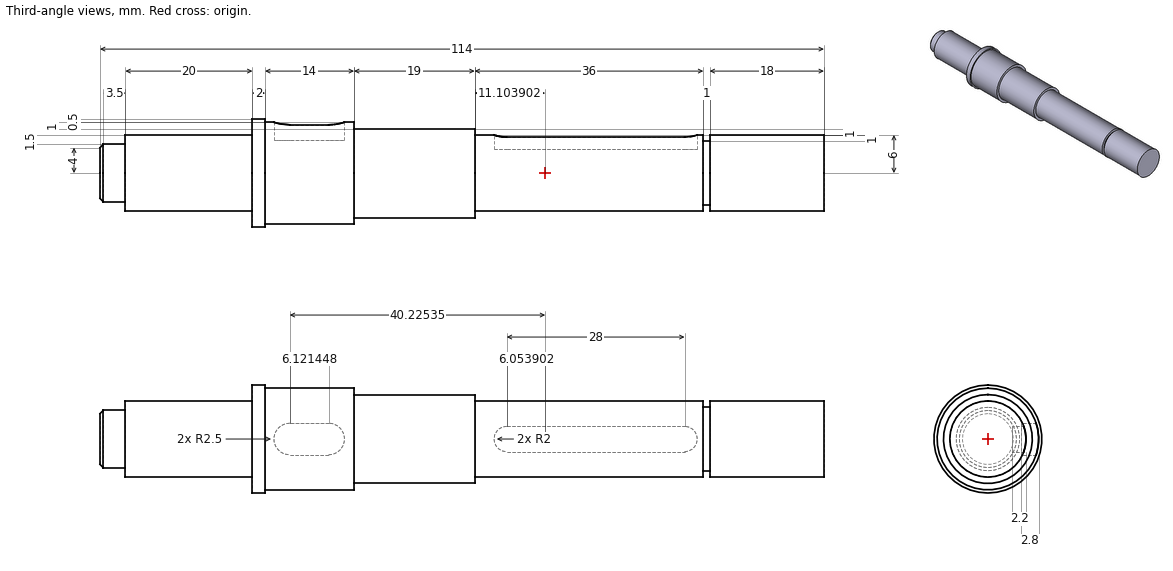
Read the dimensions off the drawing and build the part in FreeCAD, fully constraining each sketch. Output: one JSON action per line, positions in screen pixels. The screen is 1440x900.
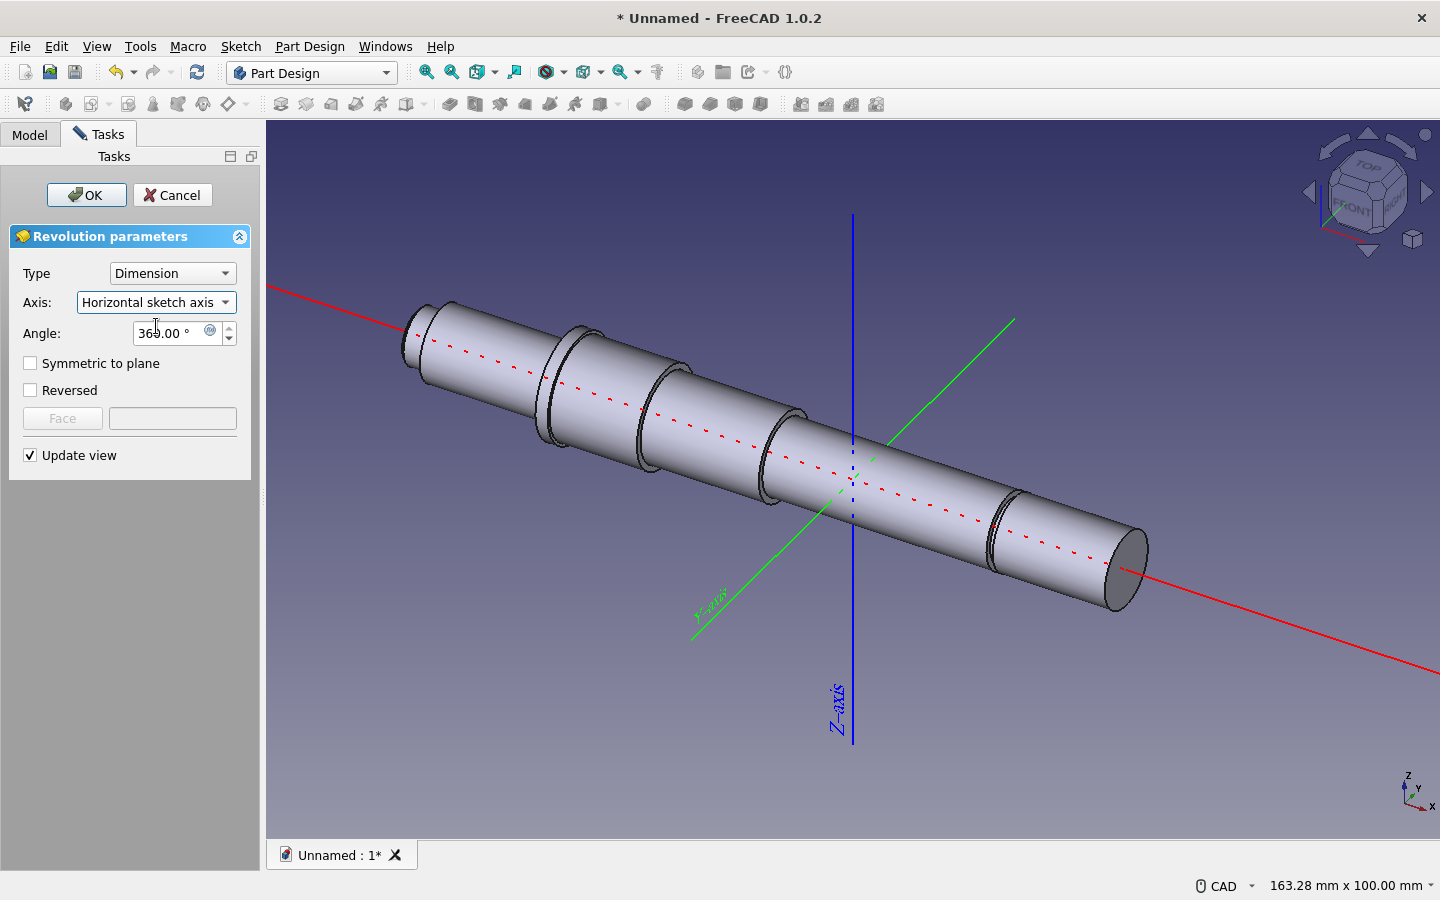
{"action": "left_click", "coordinate": [87, 195]}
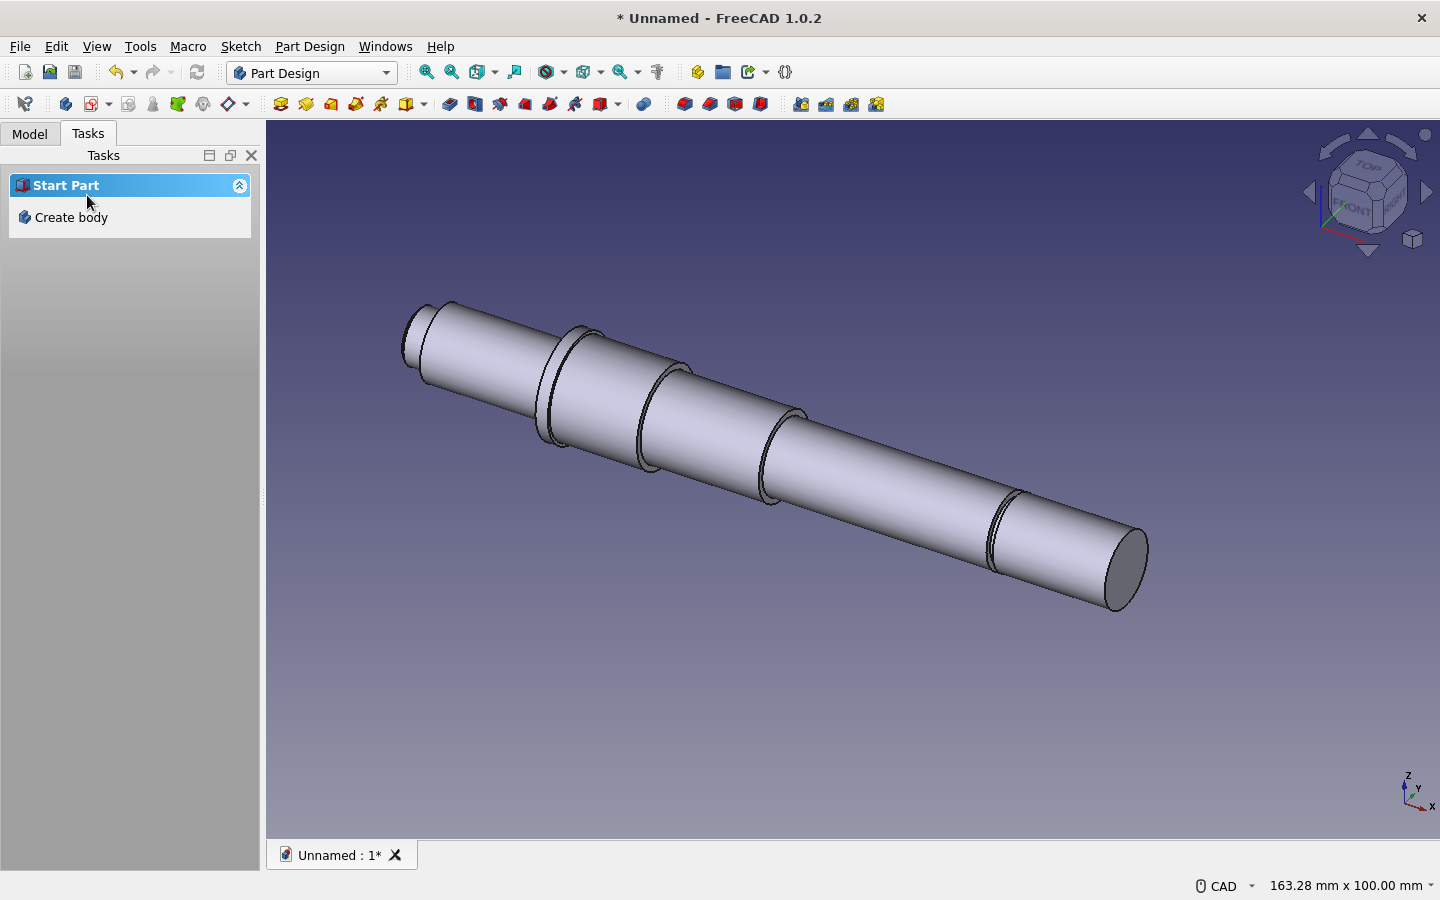
{"action": "left_click", "coordinate": [30, 134]}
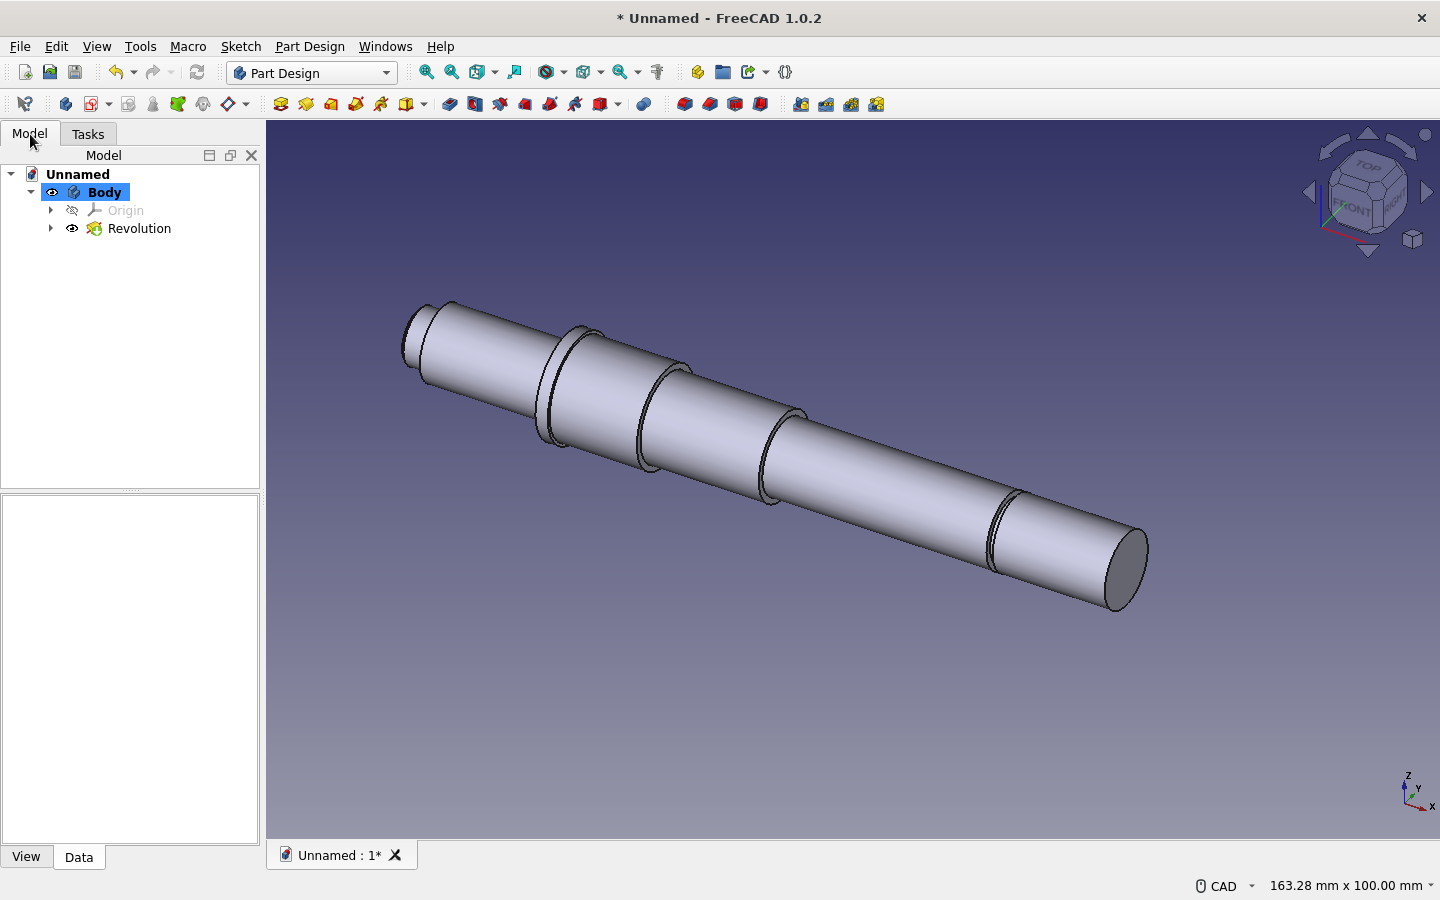
{"action": "left_click", "coordinate": [51, 210]}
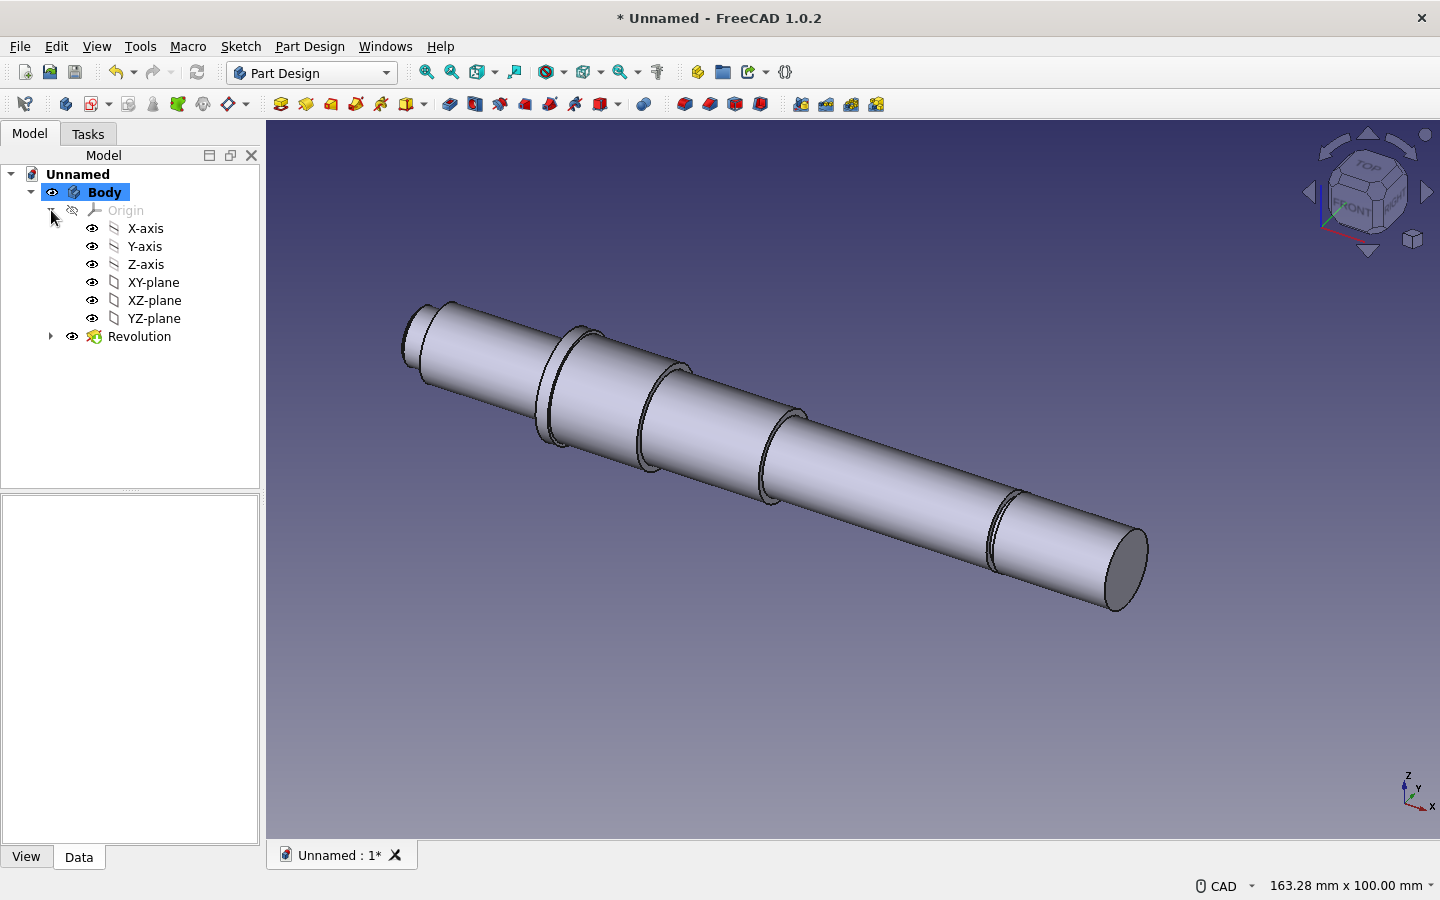
{"action": "left_click", "coordinate": [137, 300]}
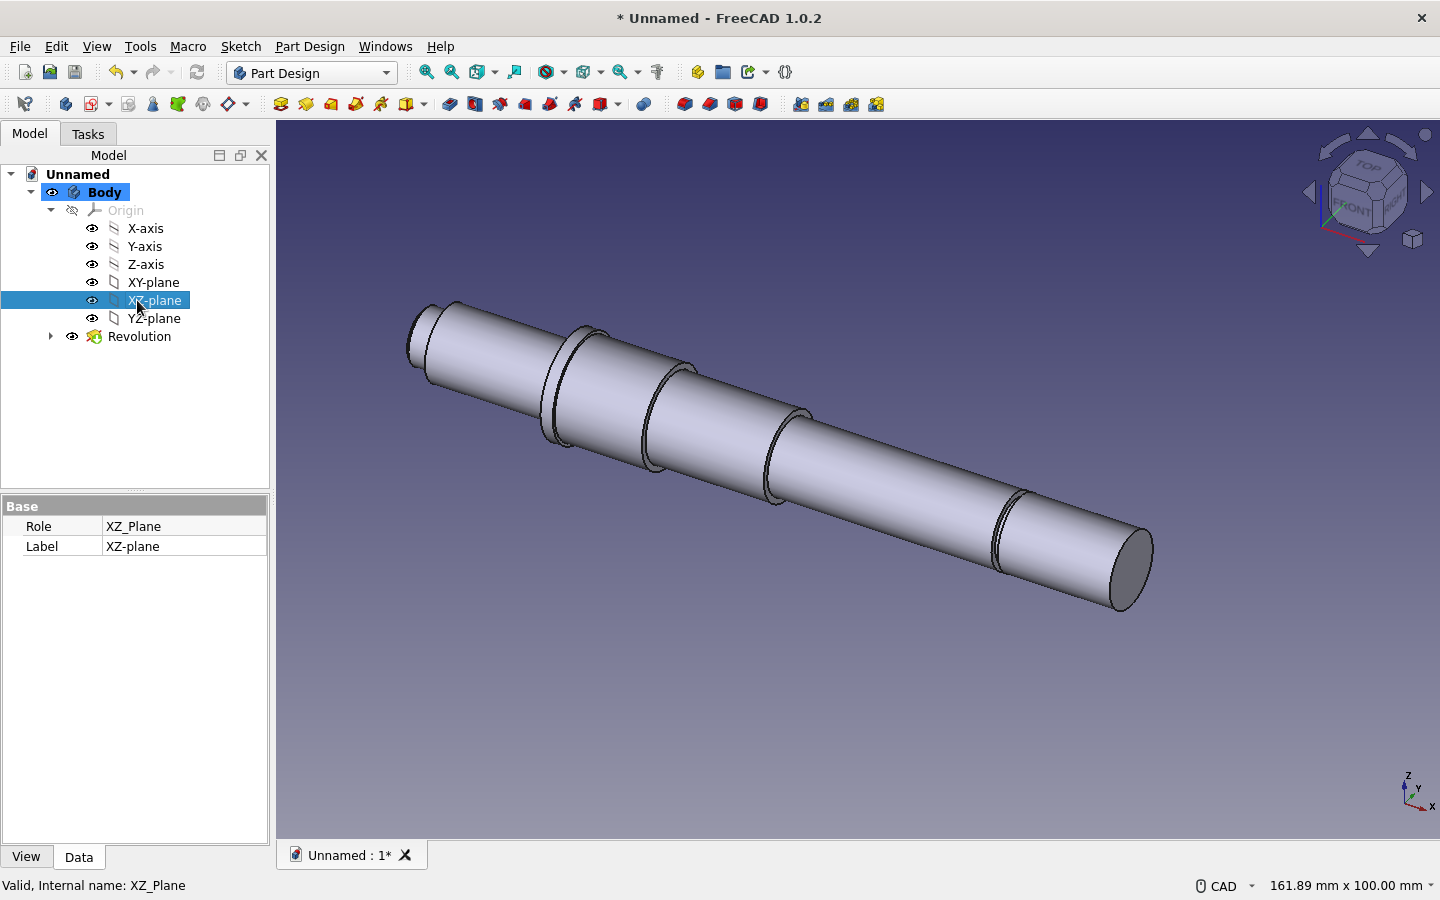
{"action": "left_click", "coordinate": [228, 104]}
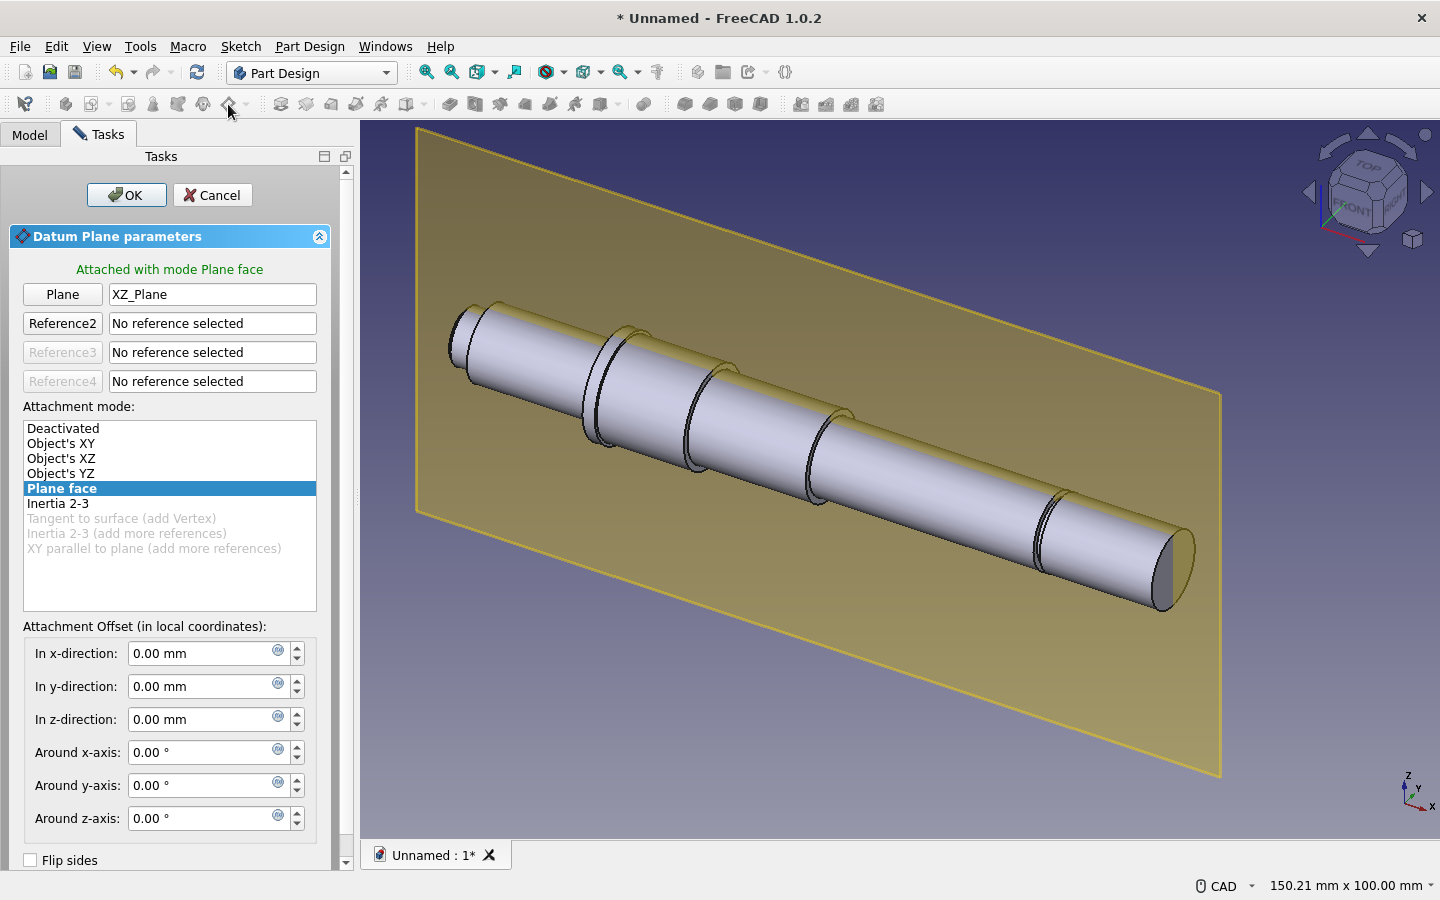
{"action": "triple_click", "coordinate": [210, 720]}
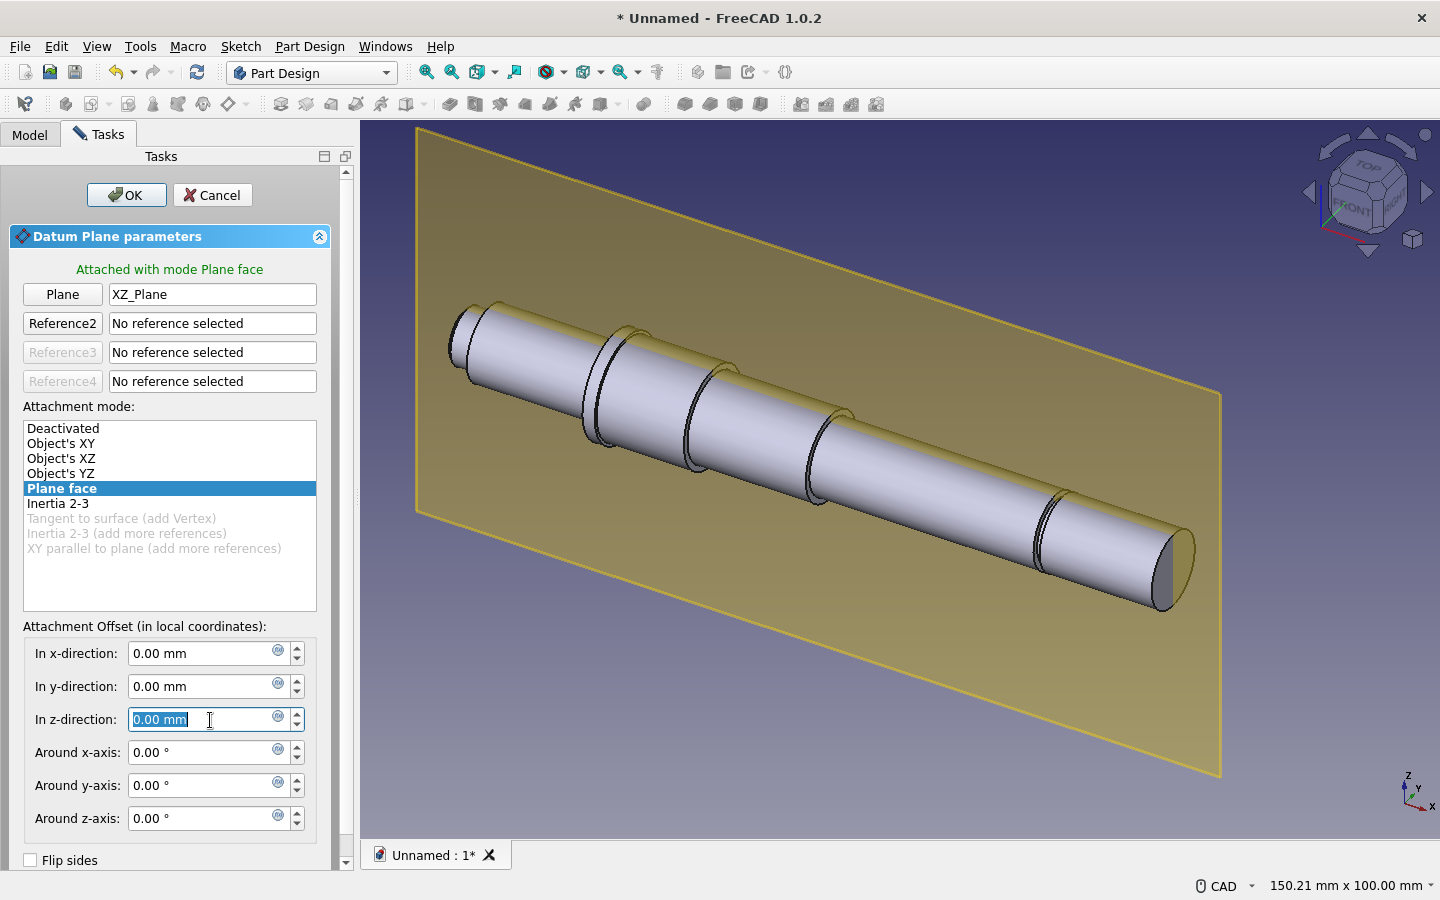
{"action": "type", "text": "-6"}
{"action": "key", "text": "Tab"}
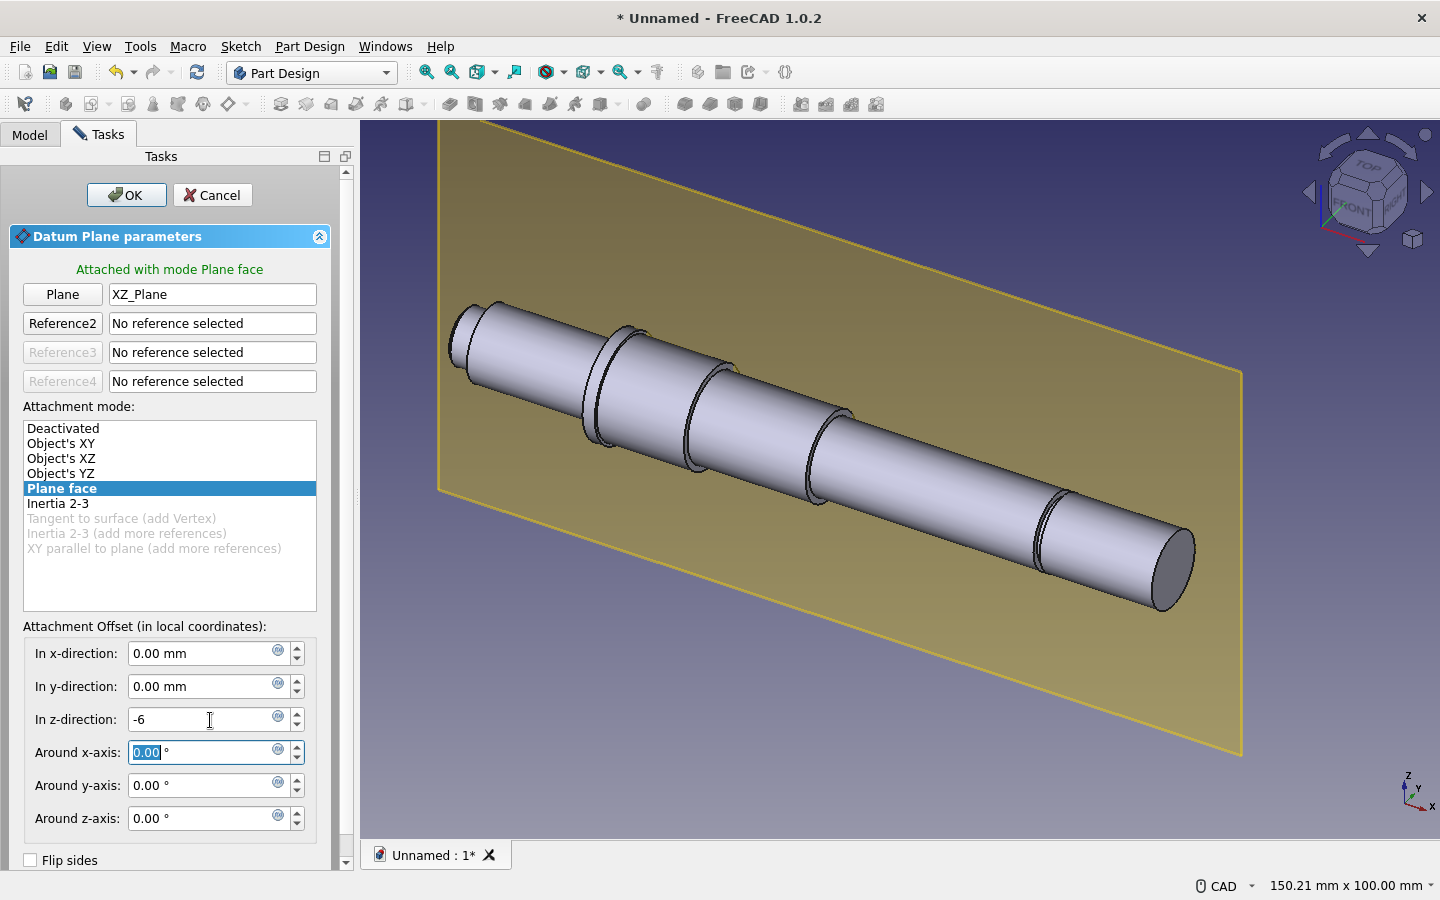
{"action": "left_click", "coordinate": [127, 195]}